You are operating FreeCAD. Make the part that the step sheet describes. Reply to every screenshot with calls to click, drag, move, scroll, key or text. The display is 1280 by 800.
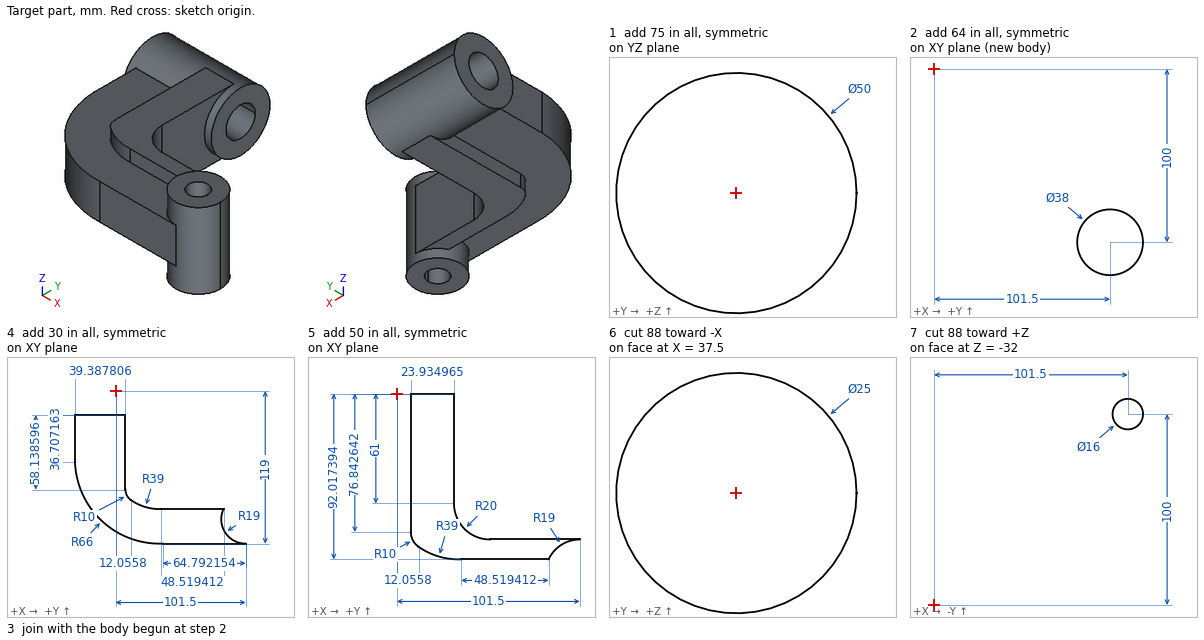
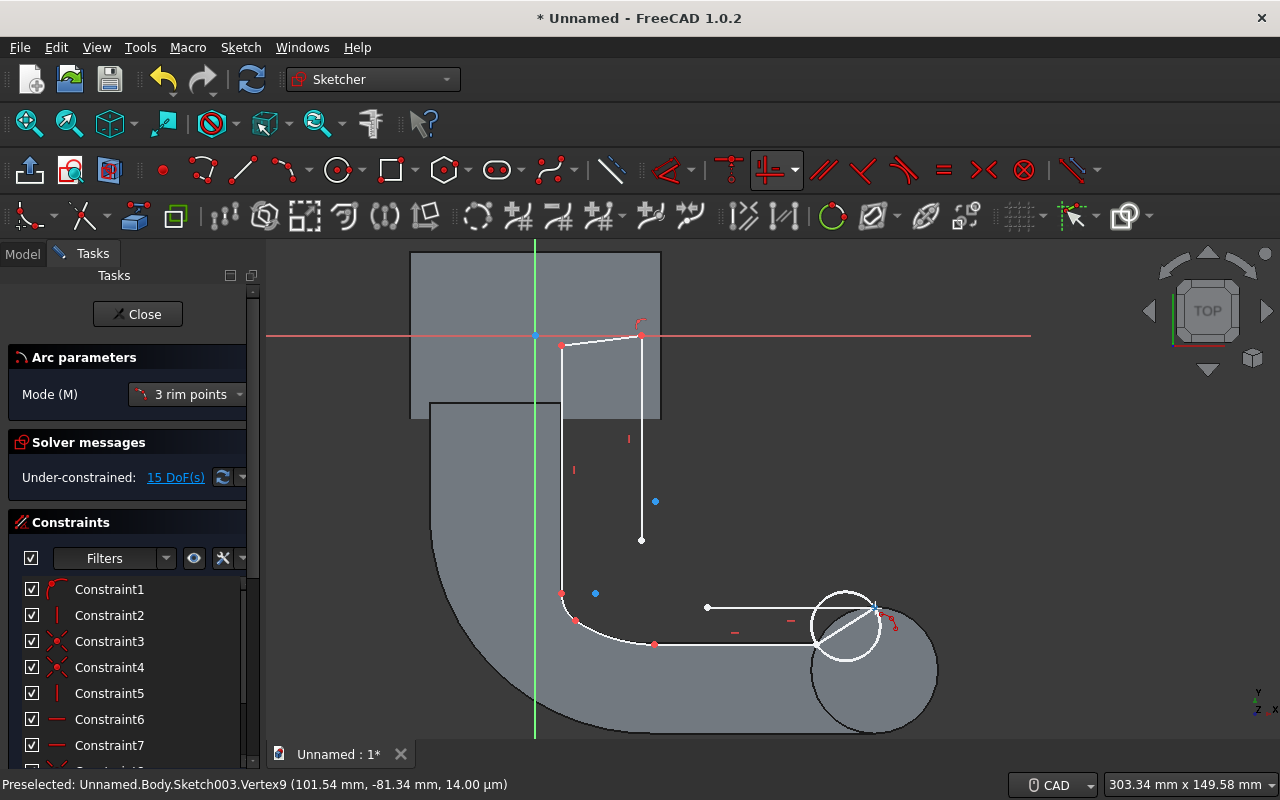
scroll(840, 617, up, 3)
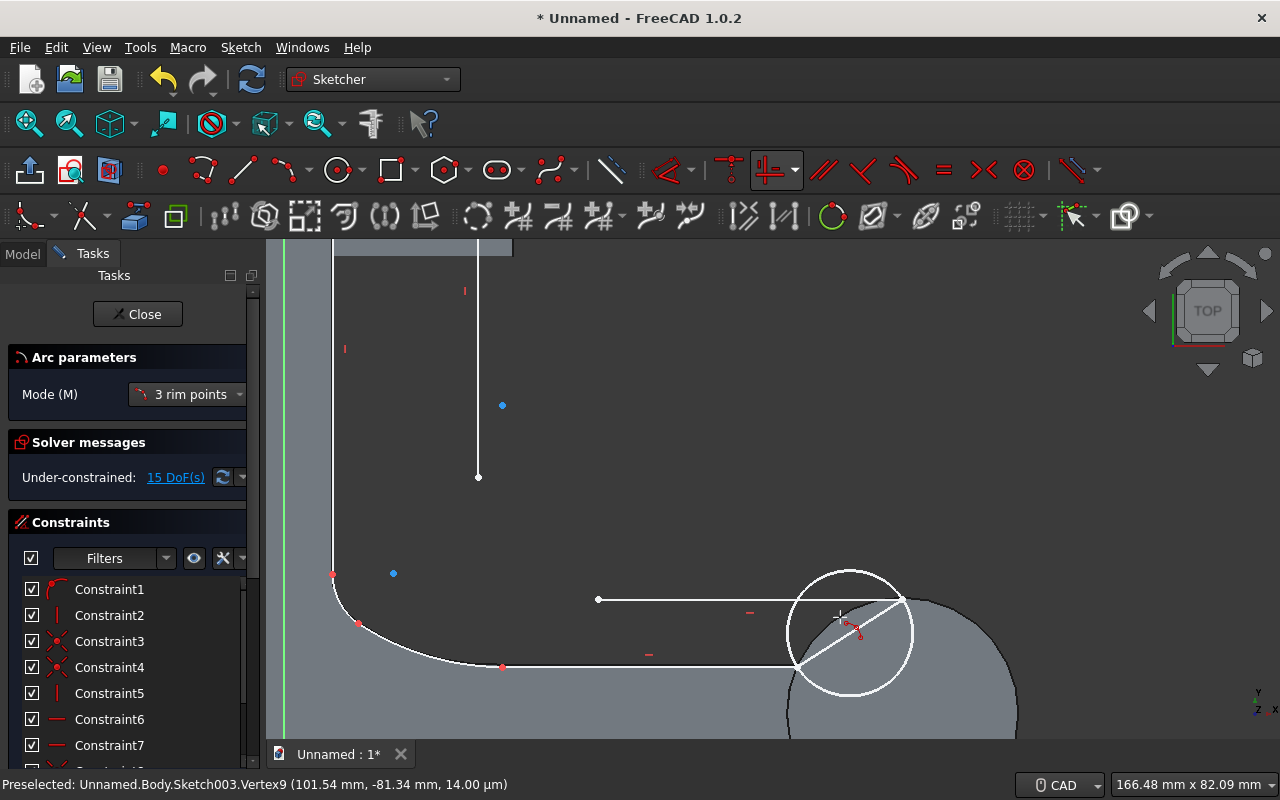
click(840, 616)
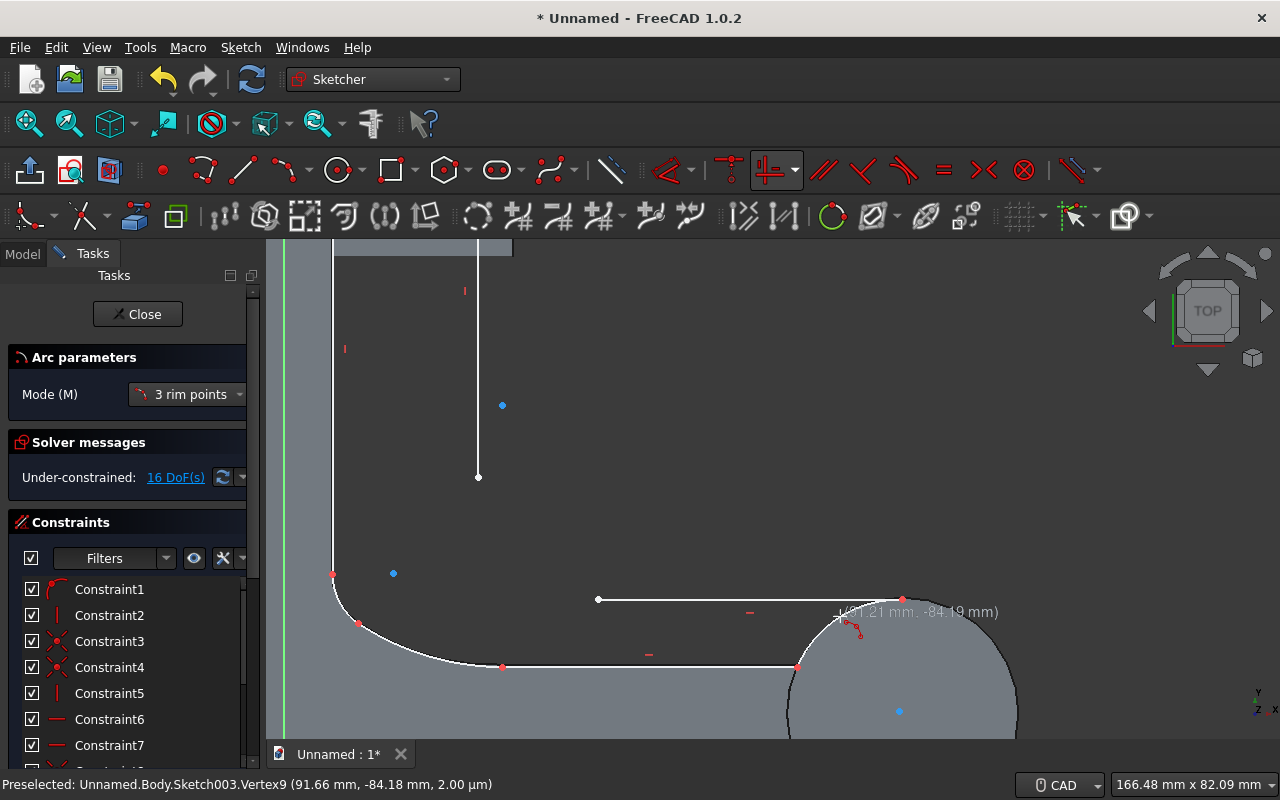
click(599, 600)
click(478, 478)
click(513, 562)
key(Escape)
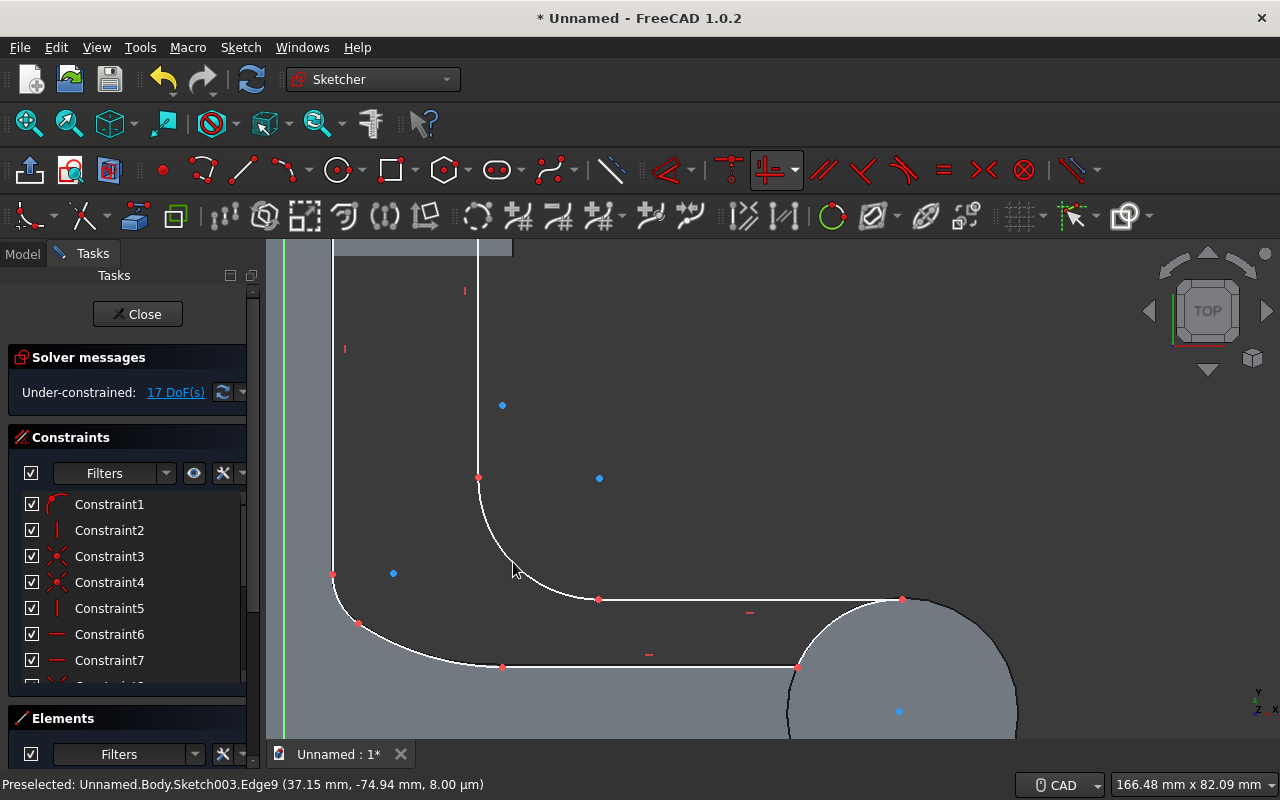
click(478, 366)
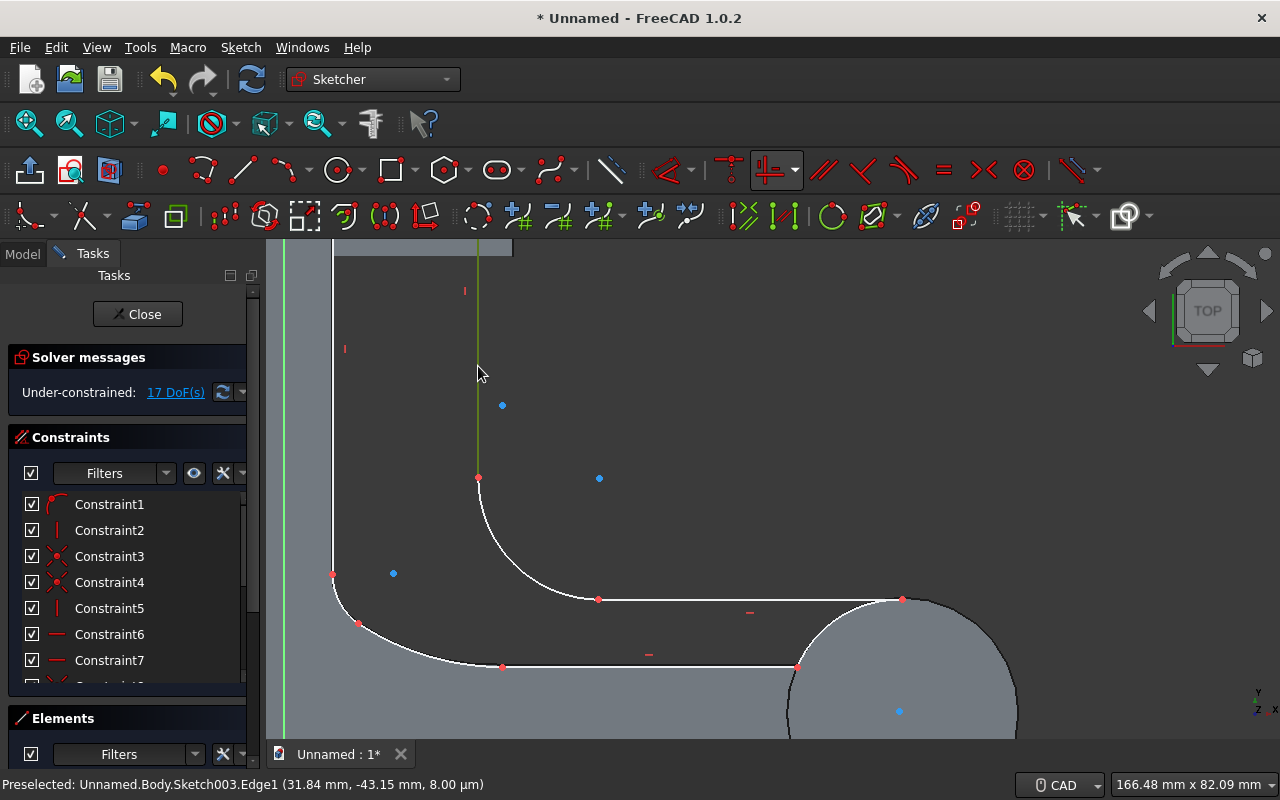
click(491, 533)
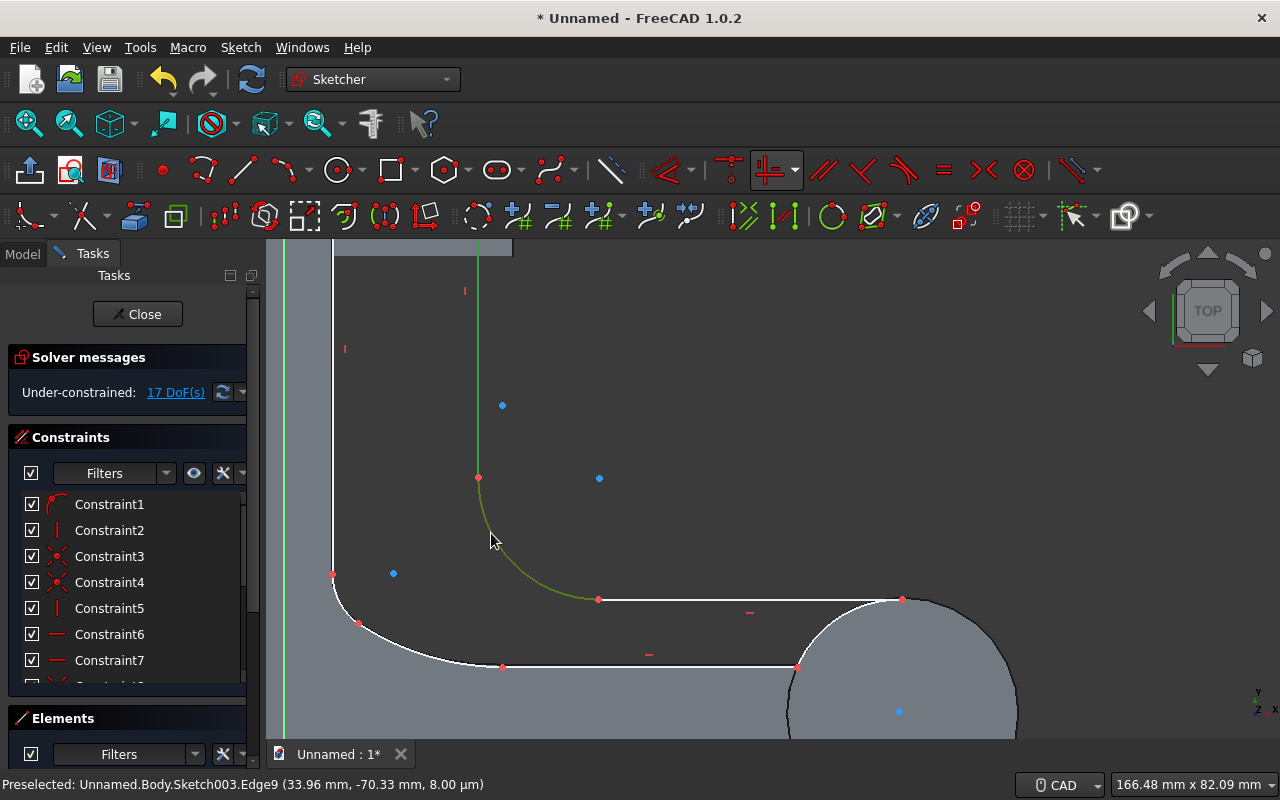
click(904, 170)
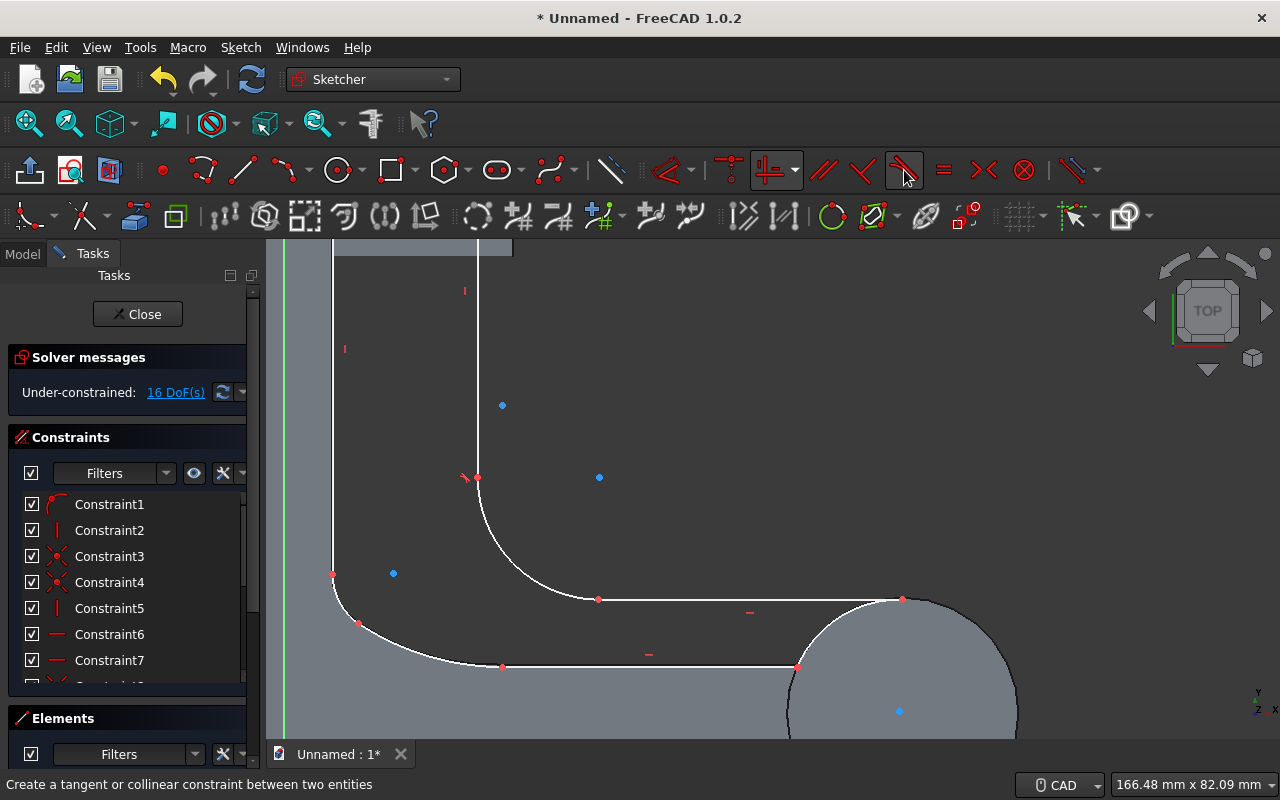
click(333, 439)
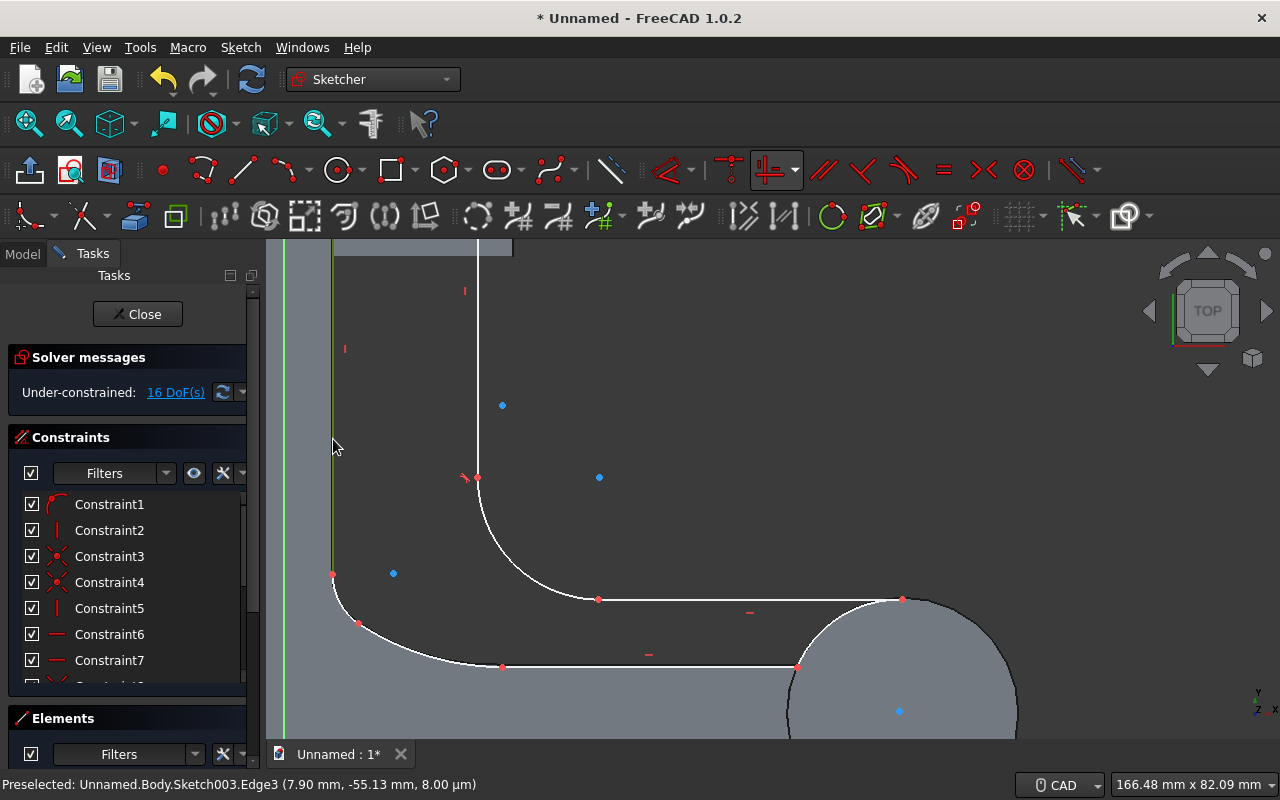
click(335, 591)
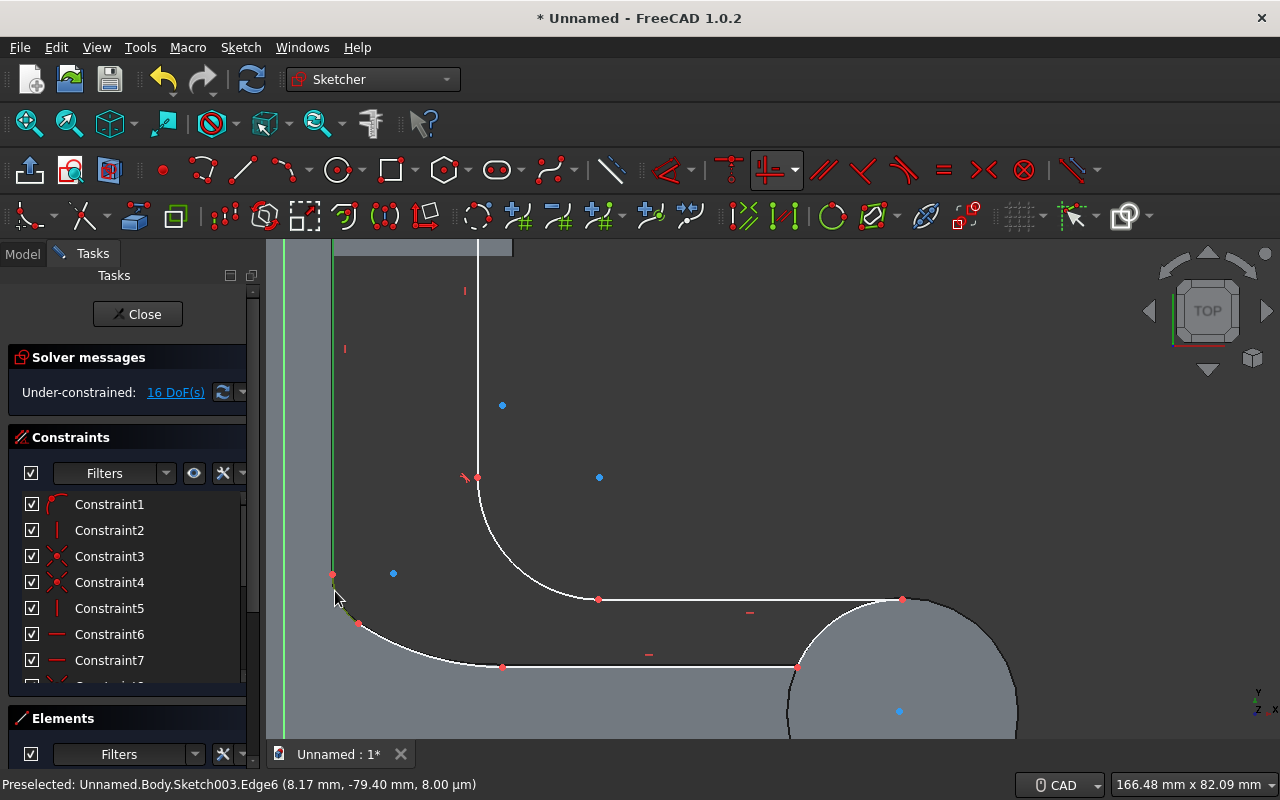
click(904, 170)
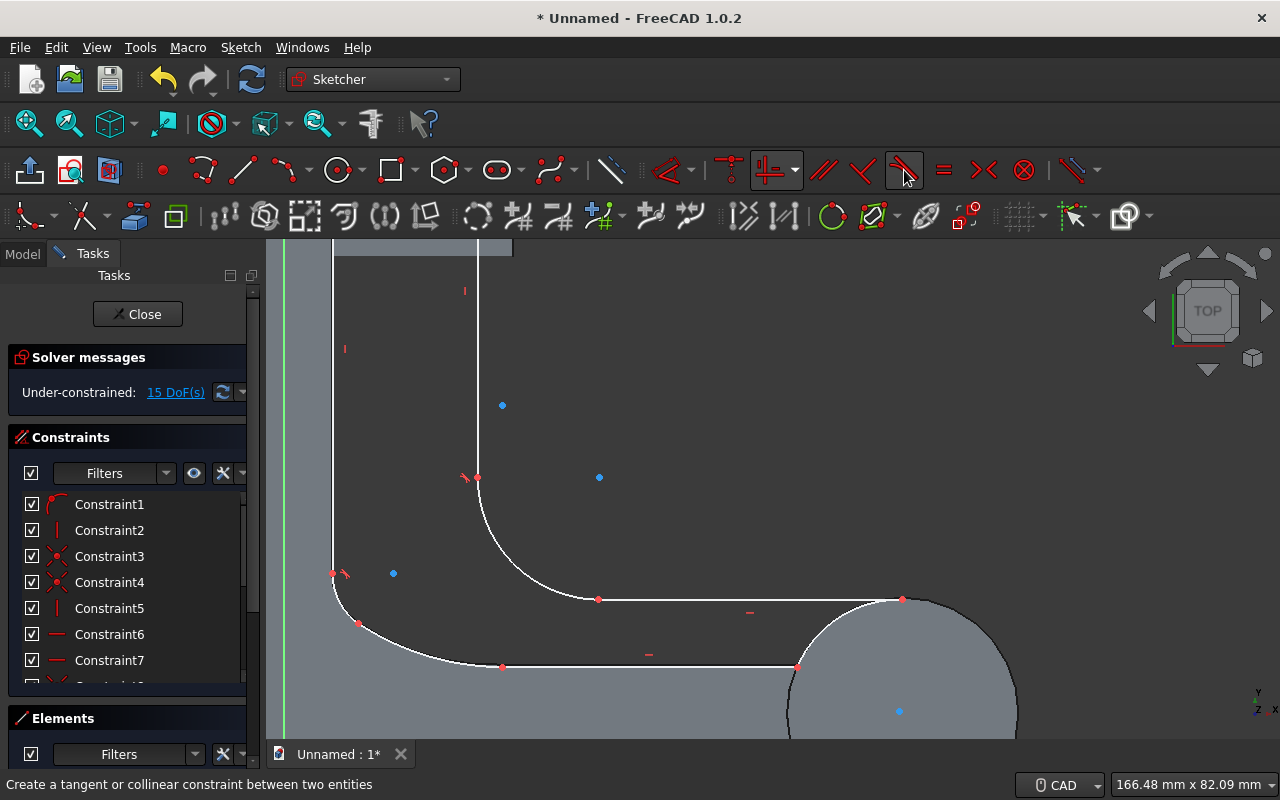
click(812, 600)